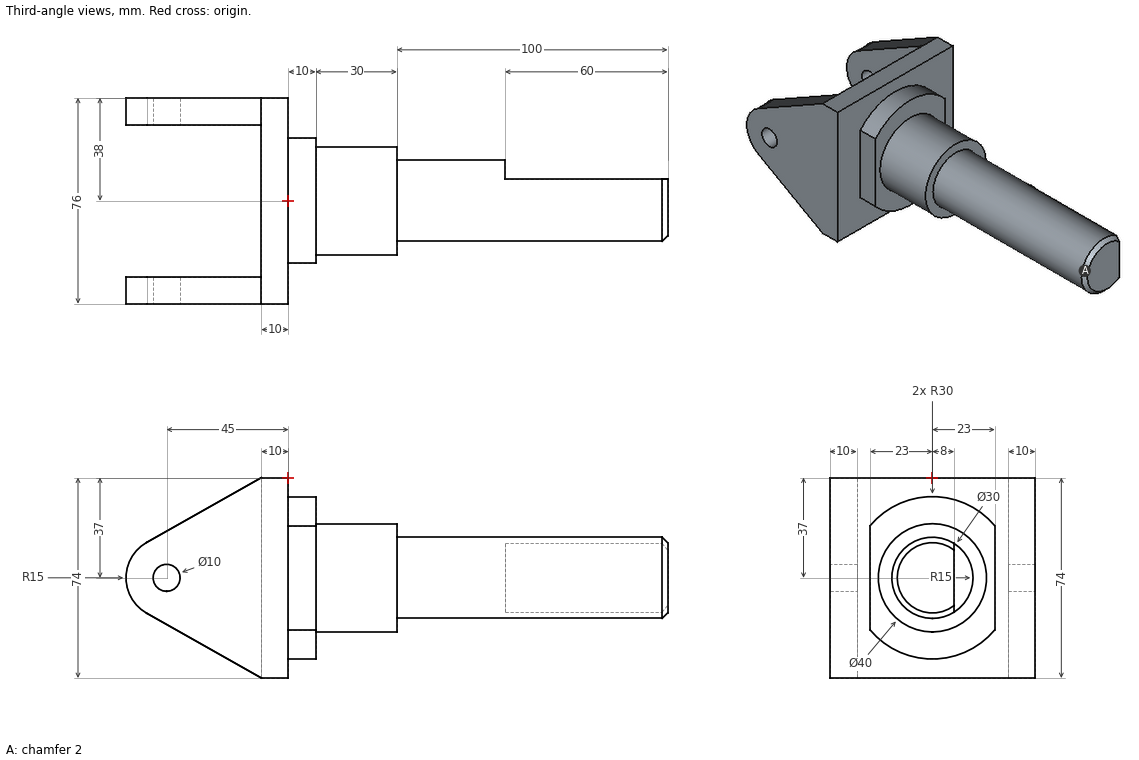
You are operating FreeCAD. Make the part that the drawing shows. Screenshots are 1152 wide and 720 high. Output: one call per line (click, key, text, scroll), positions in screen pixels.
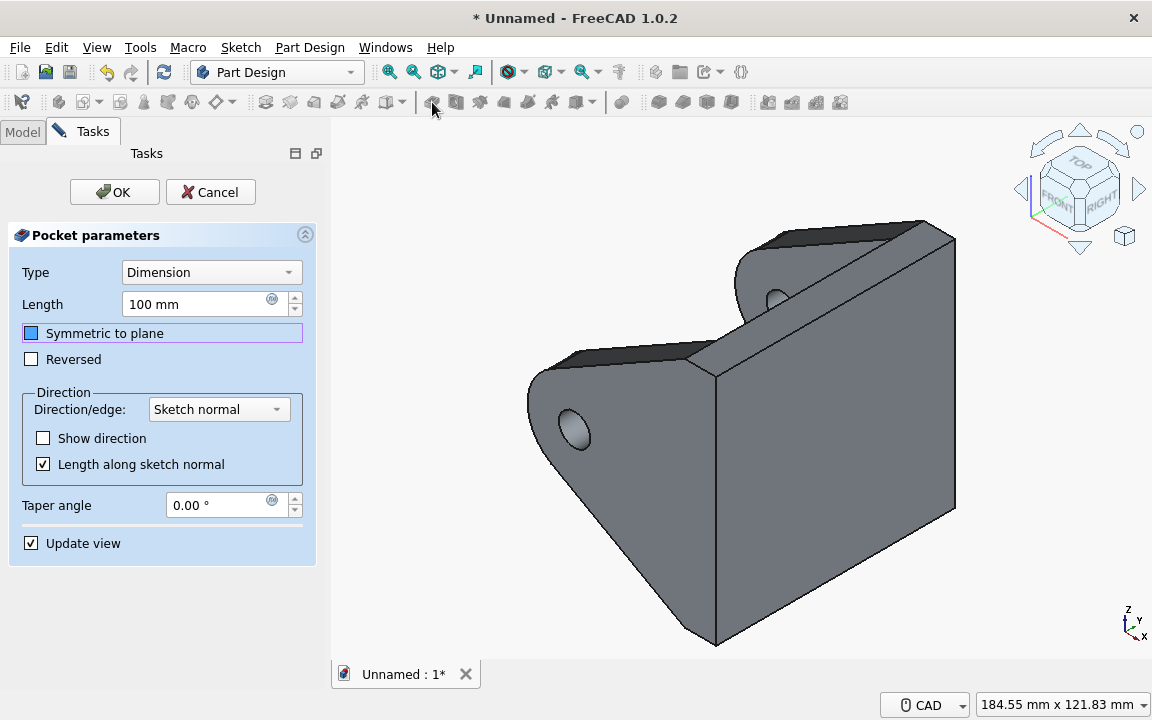
click(115, 192)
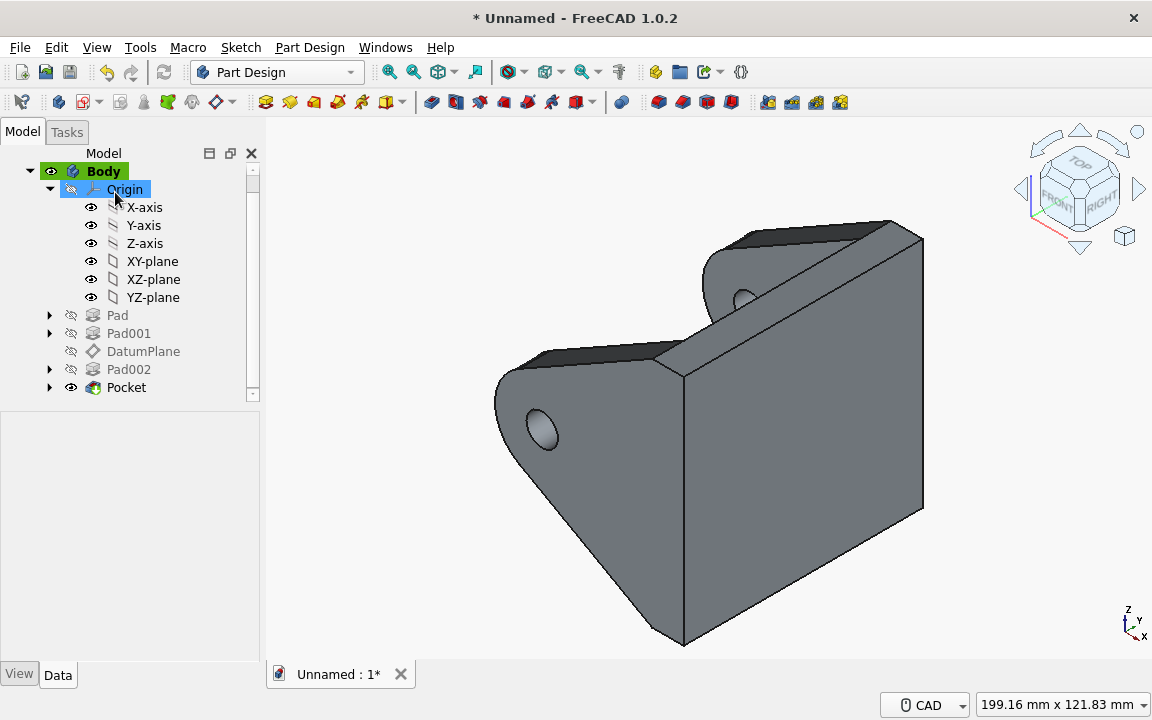
click(84, 102)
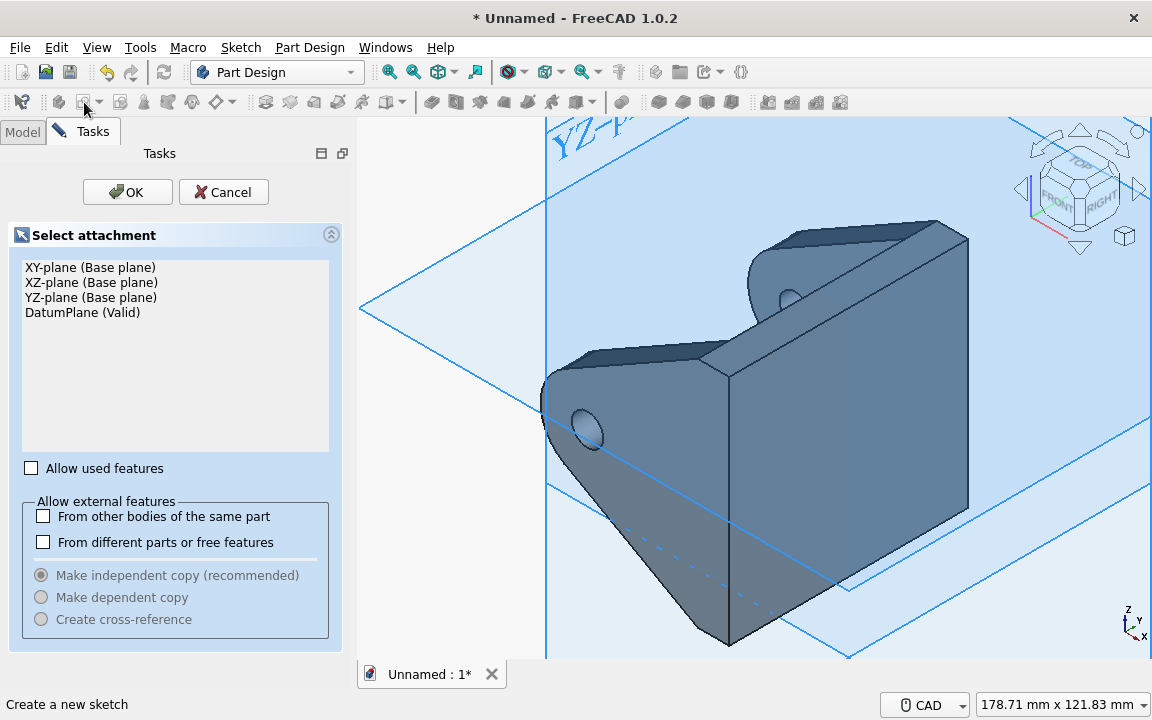
click(82, 298)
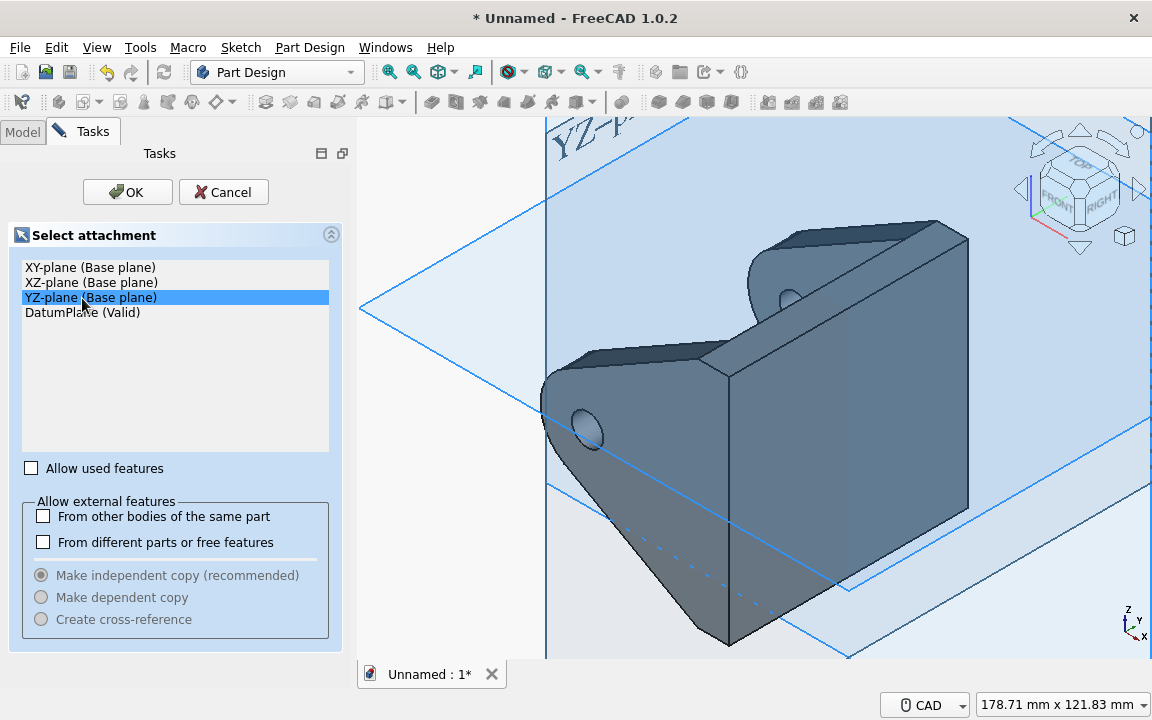
click(128, 192)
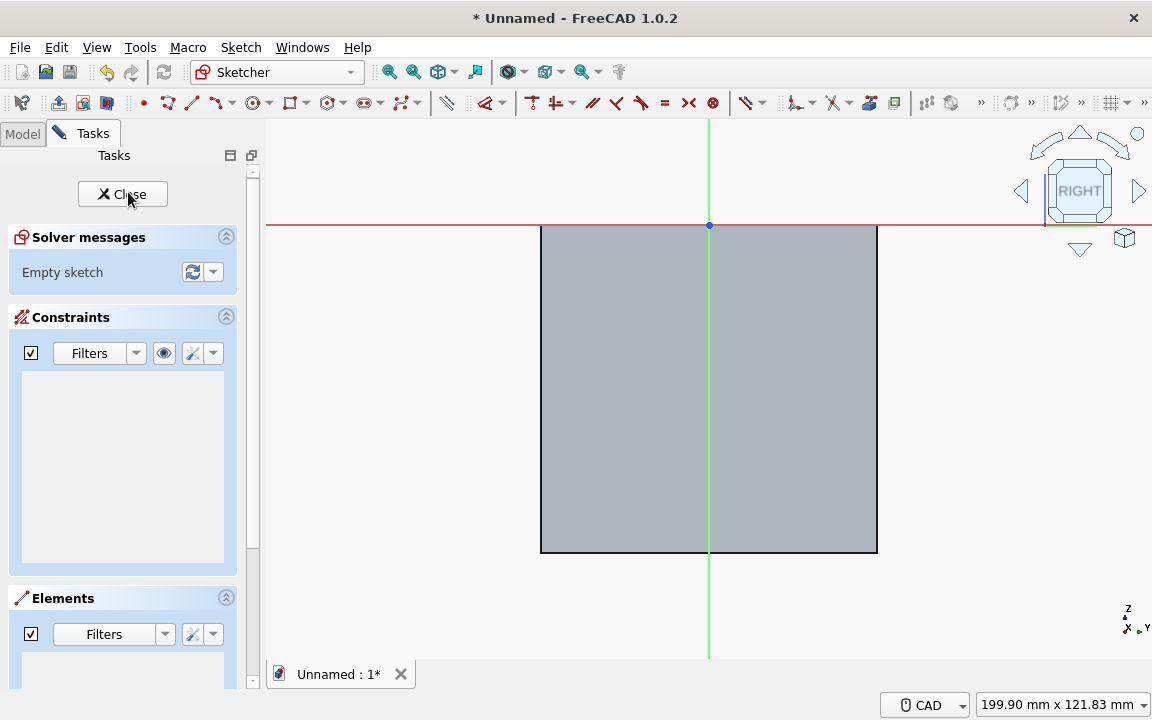
click(192, 104)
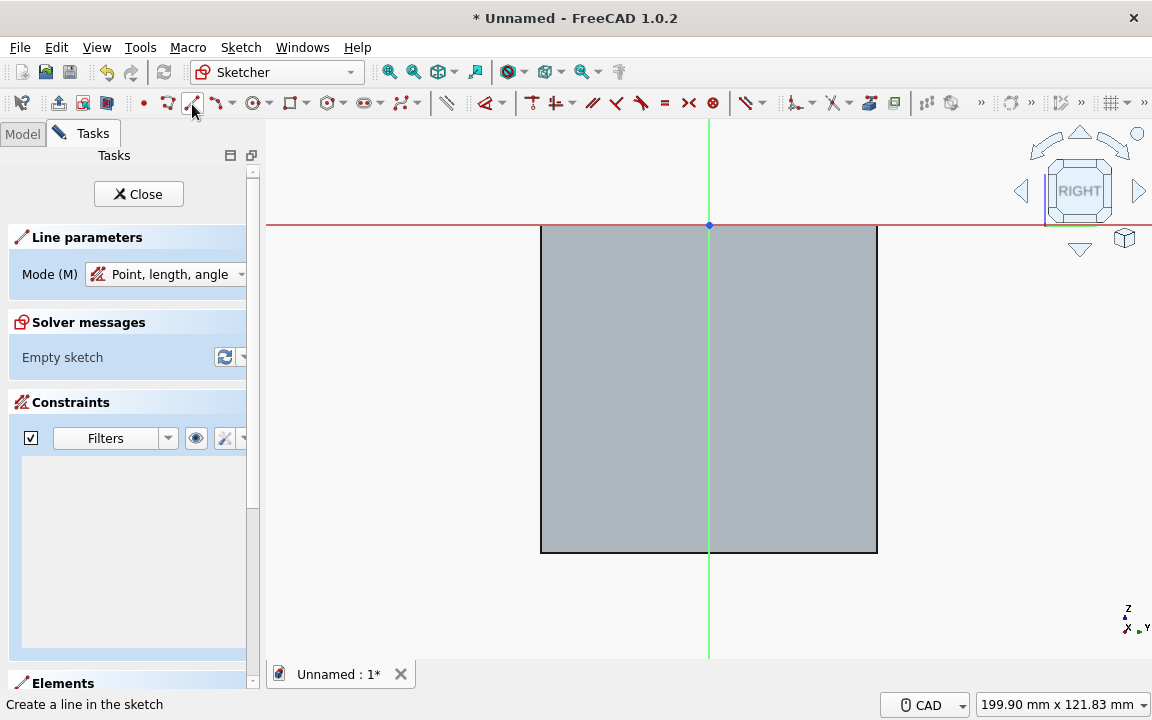
click(811, 474)
click(811, 304)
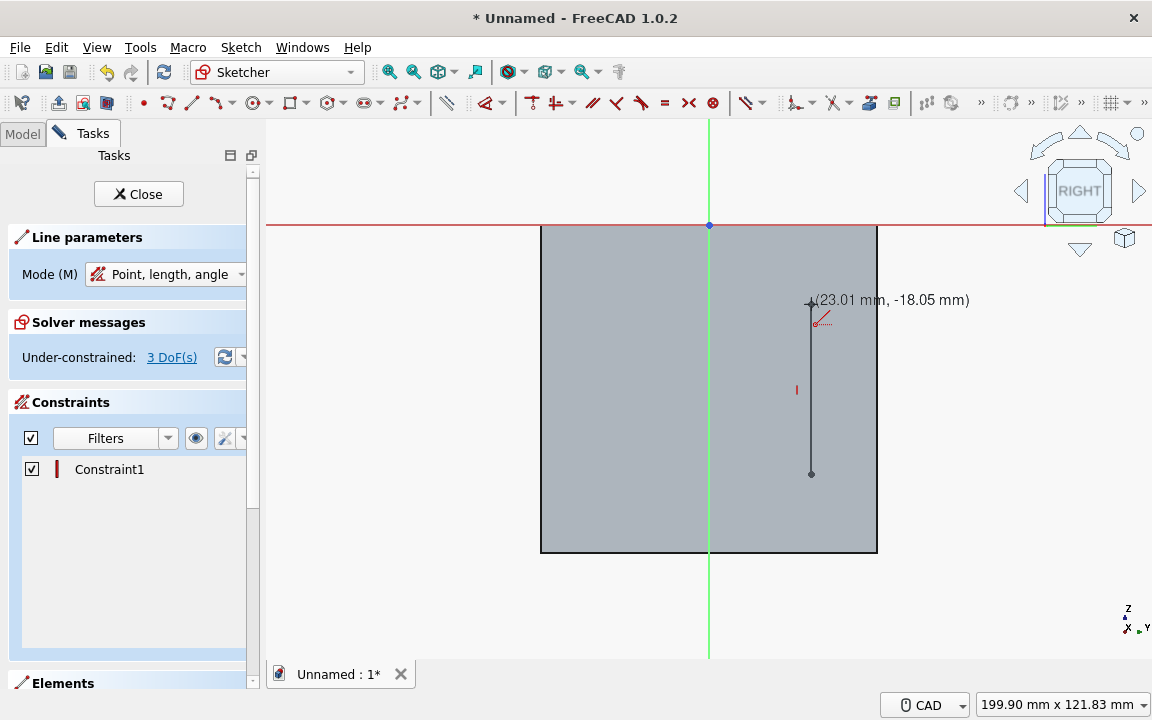
click(607, 304)
click(607, 474)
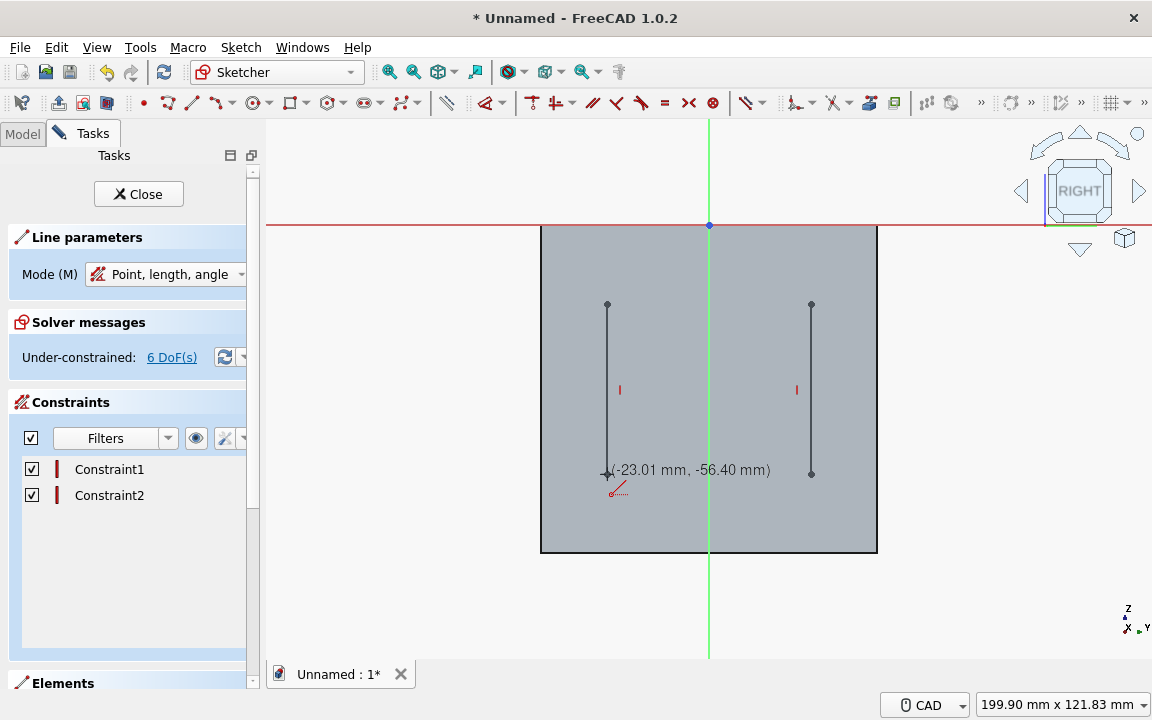
click(216, 104)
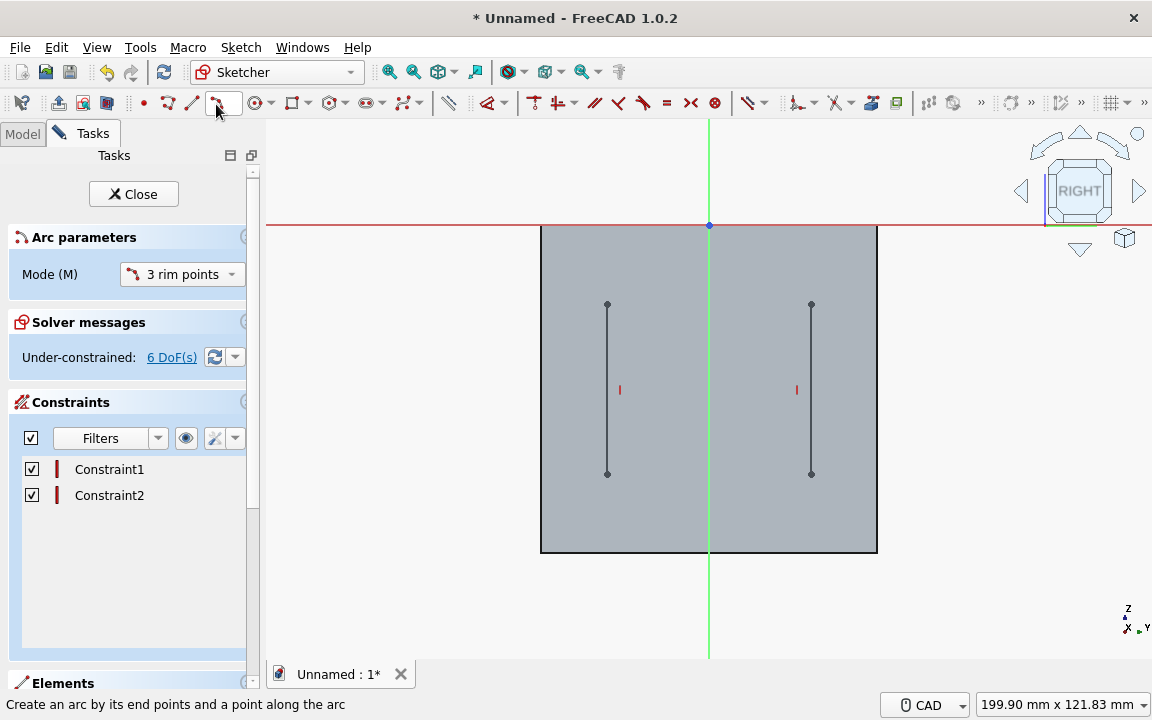
click(811, 305)
click(607, 305)
click(732, 258)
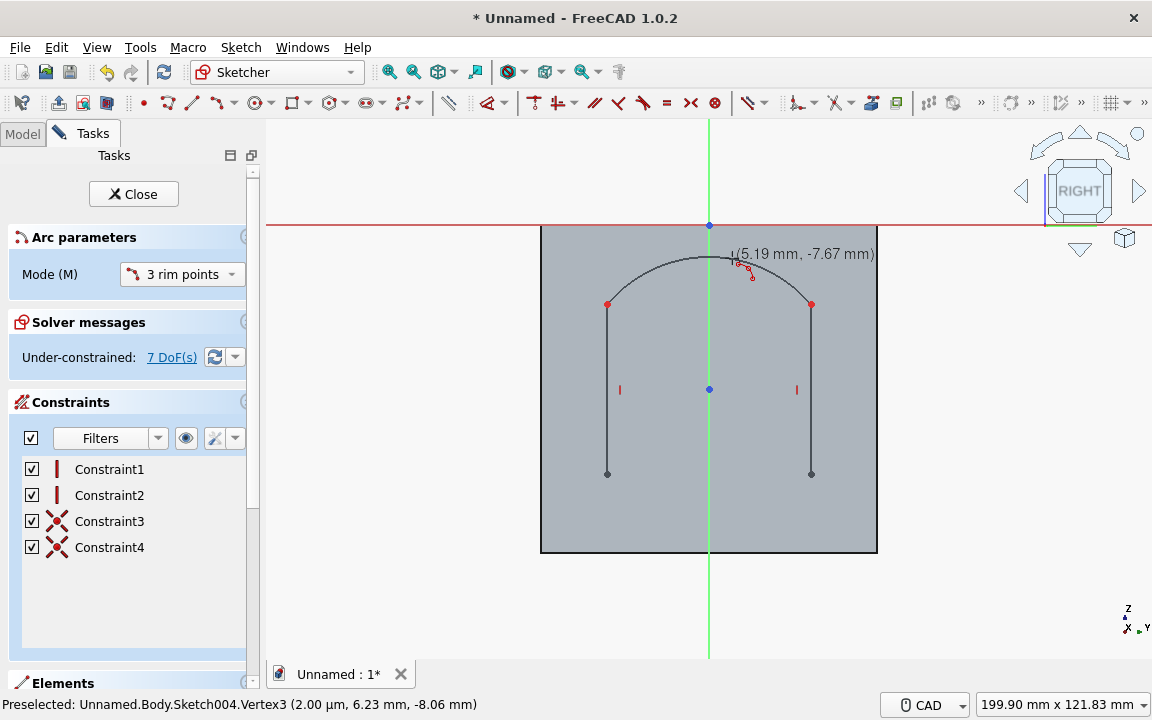
click(607, 475)
click(811, 475)
click(686, 520)
key(Escape)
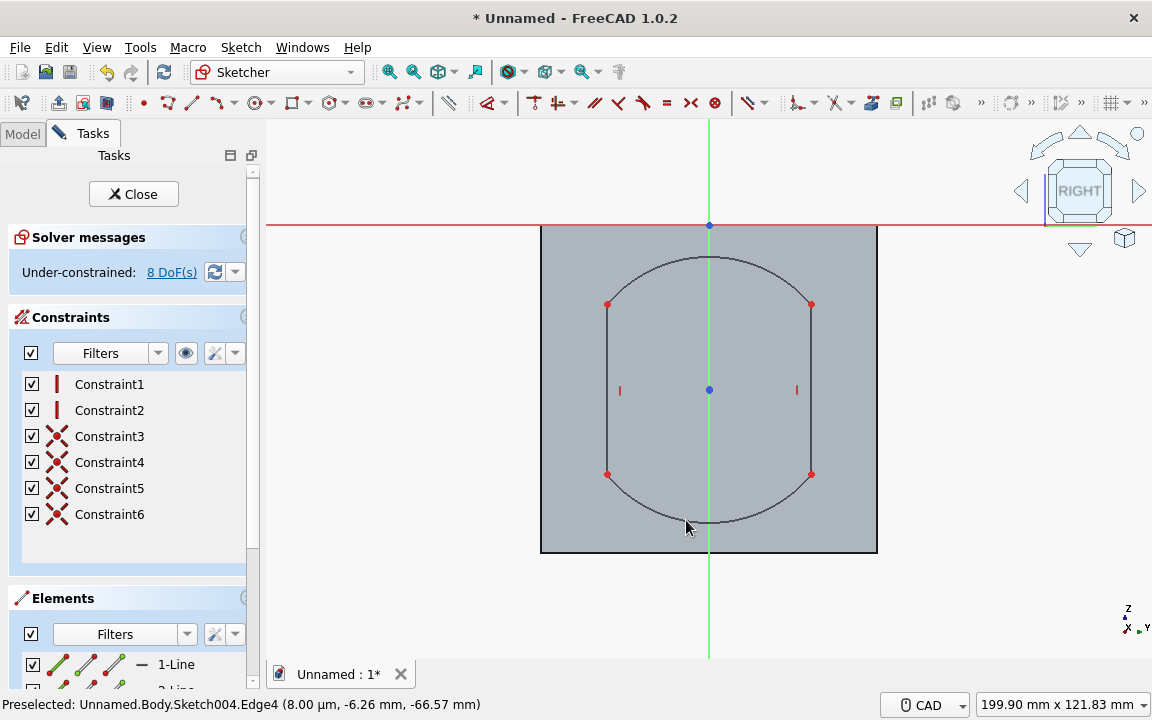
click(755, 265)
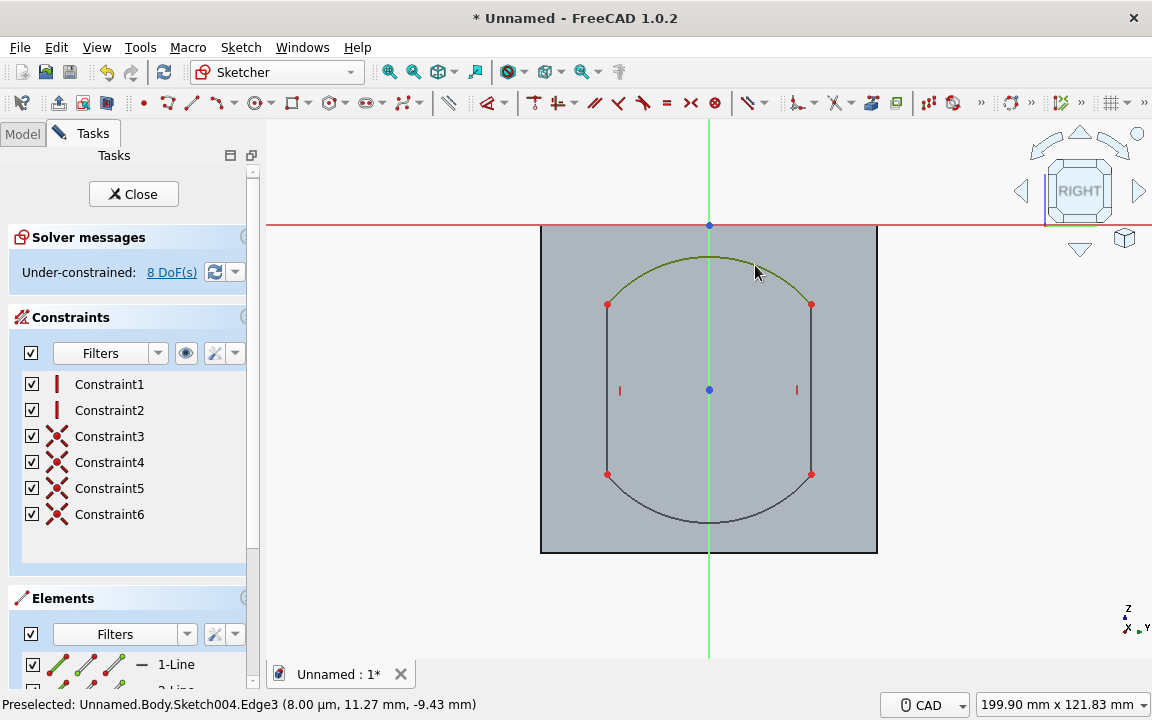
click(663, 515)